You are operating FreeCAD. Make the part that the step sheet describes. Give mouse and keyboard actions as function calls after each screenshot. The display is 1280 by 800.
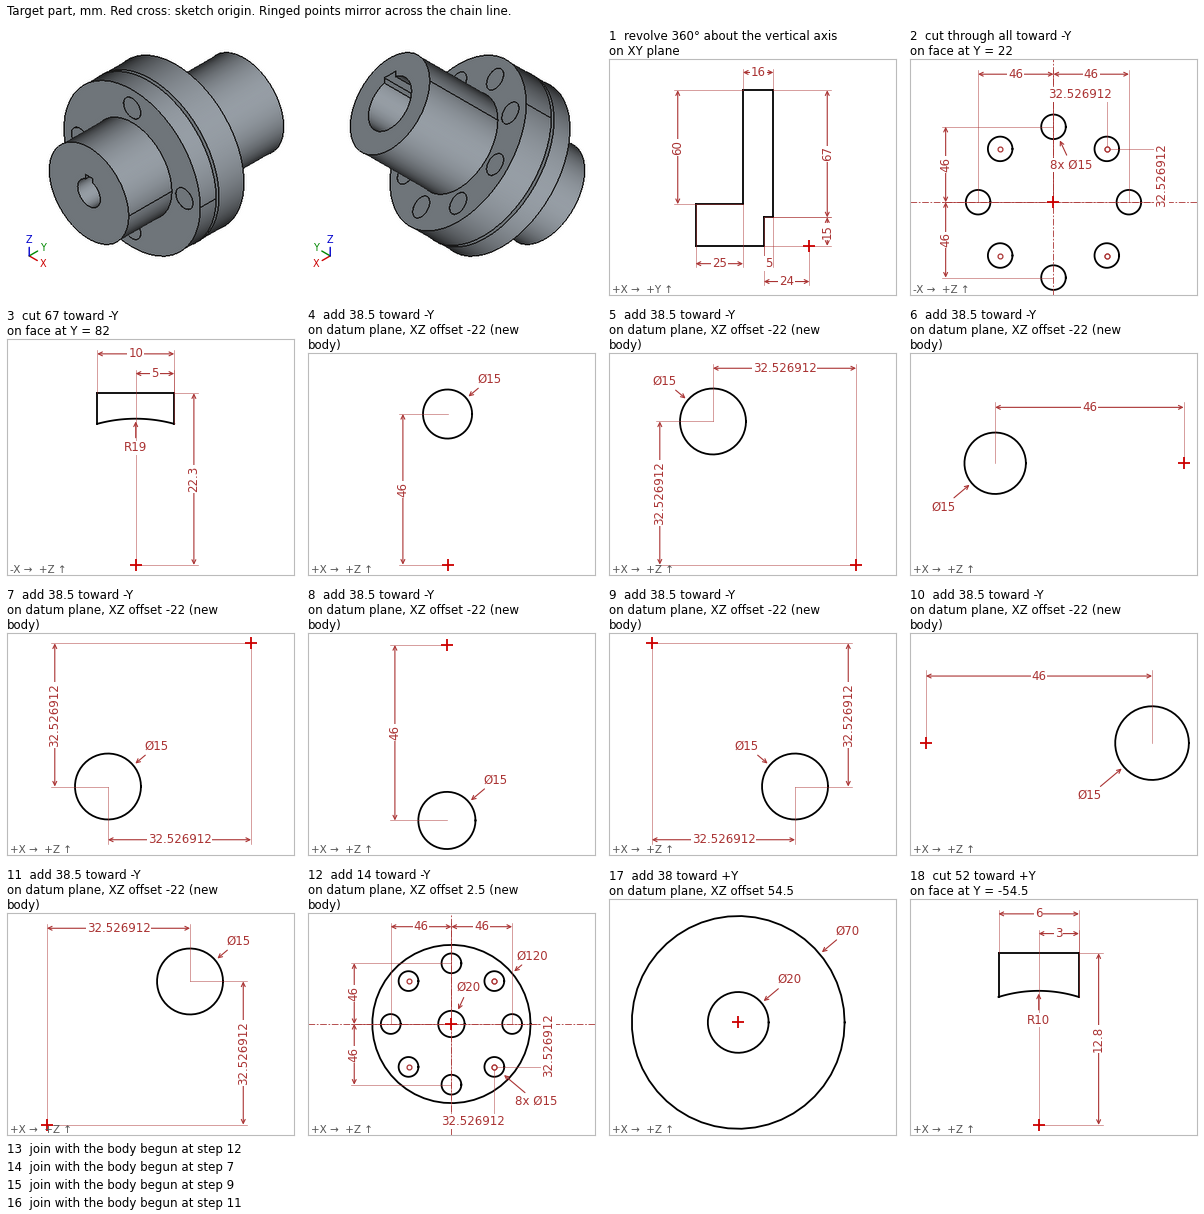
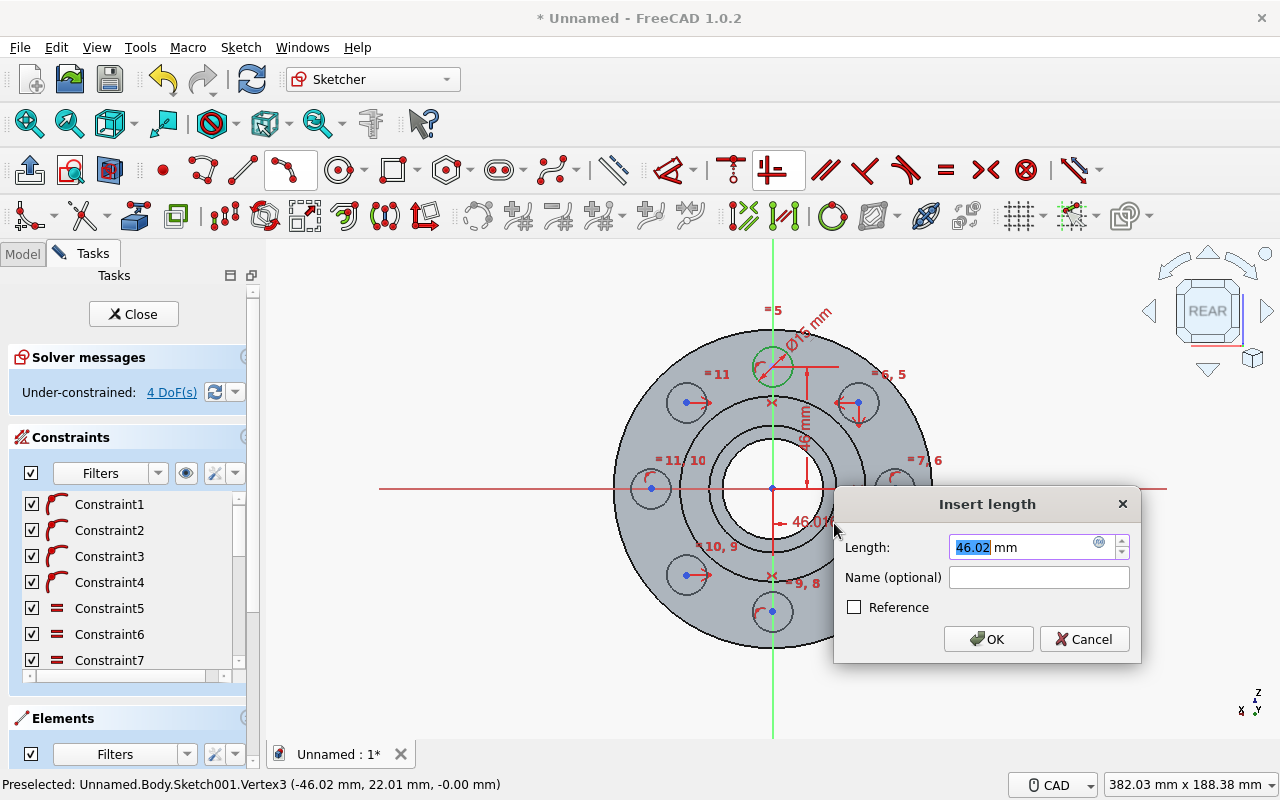
text(46)
key(Return)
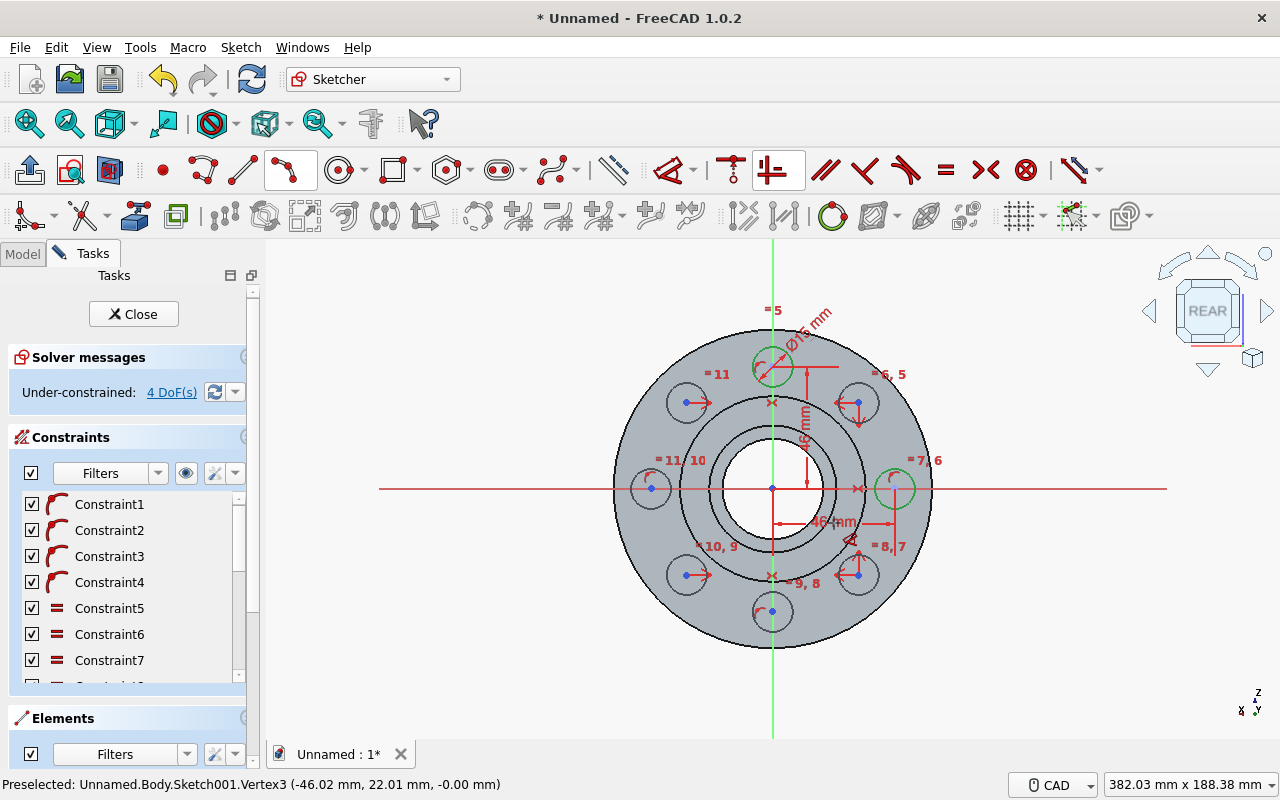
click(773, 612)
click(807, 550)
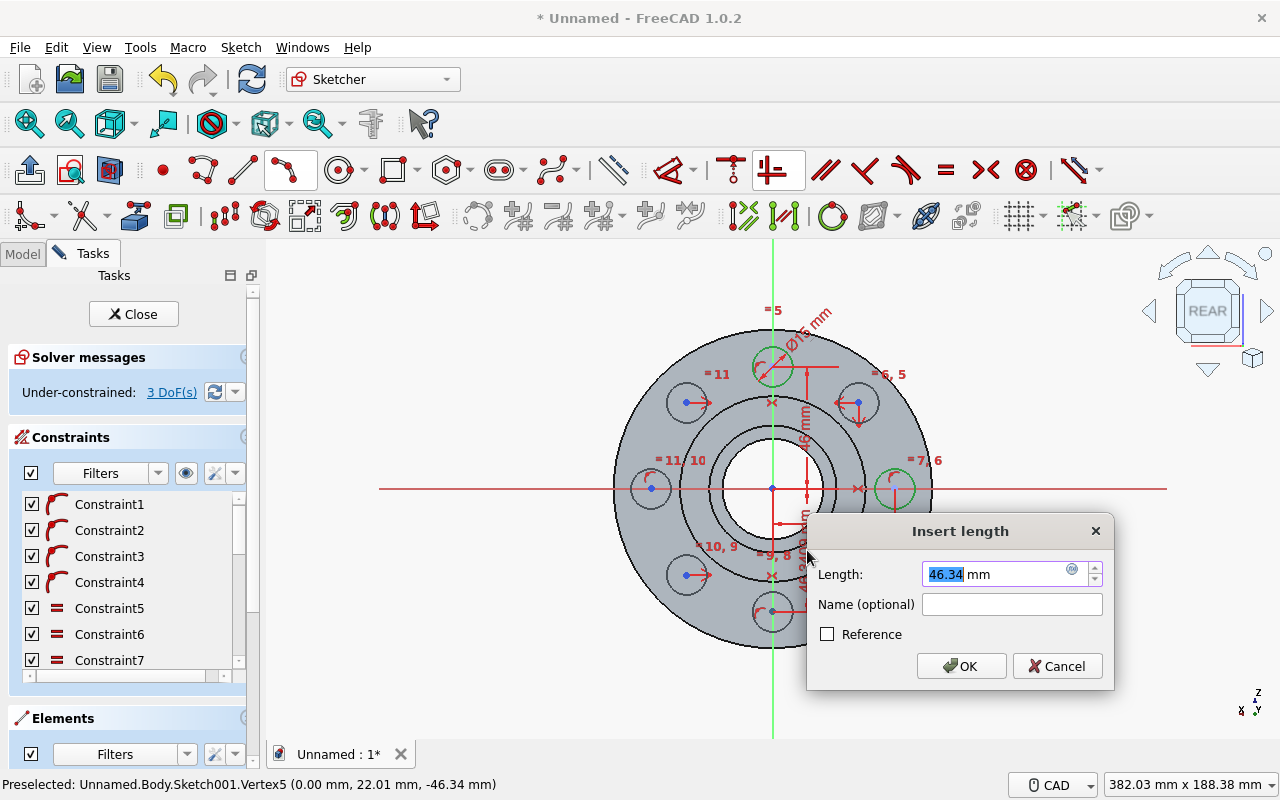
text(46)
key(Return)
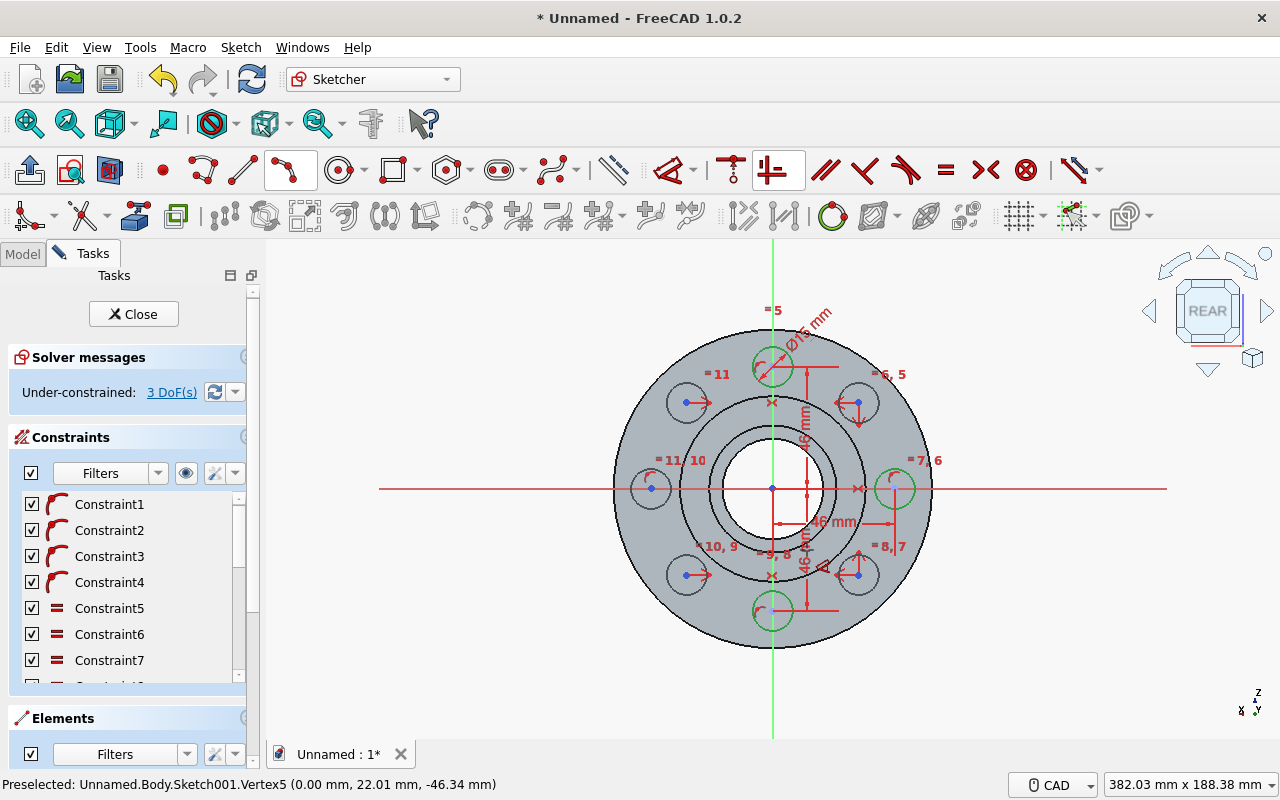
click(651, 489)
click(712, 523)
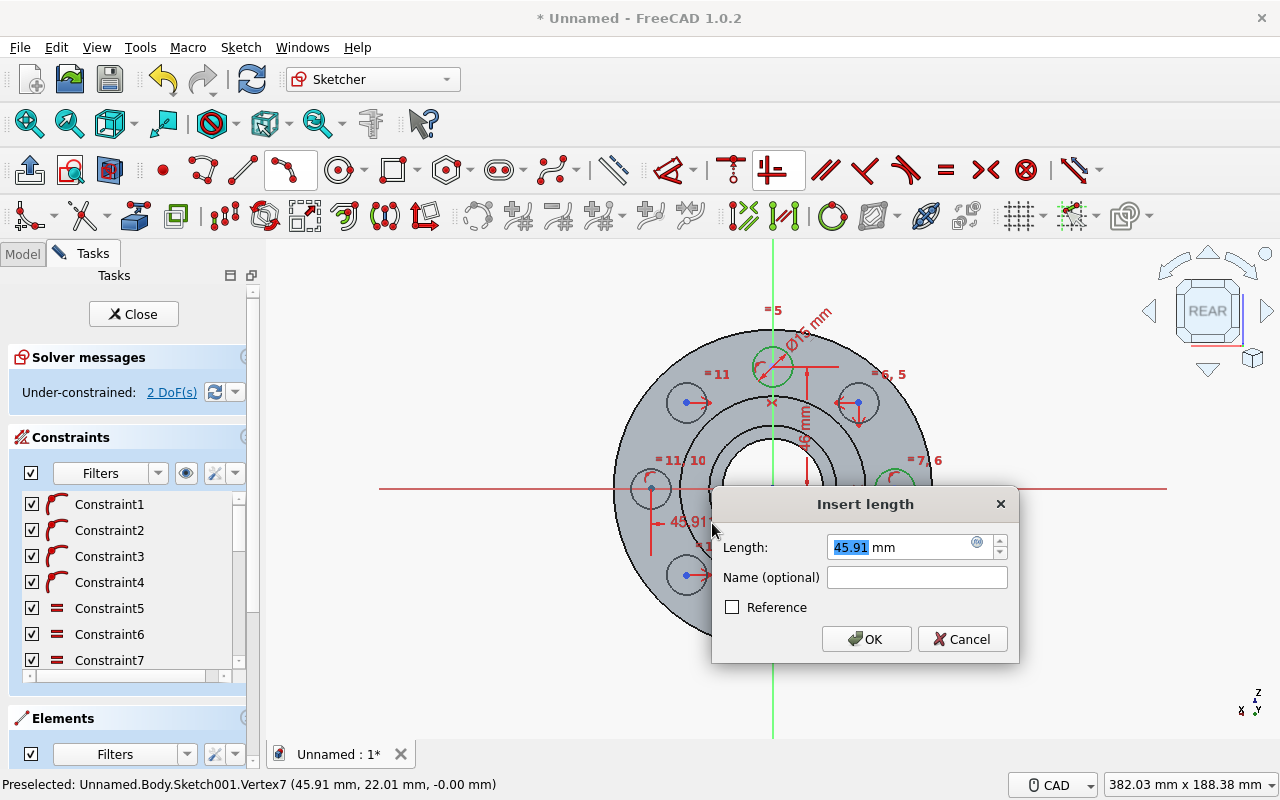
text(46)
key(Return)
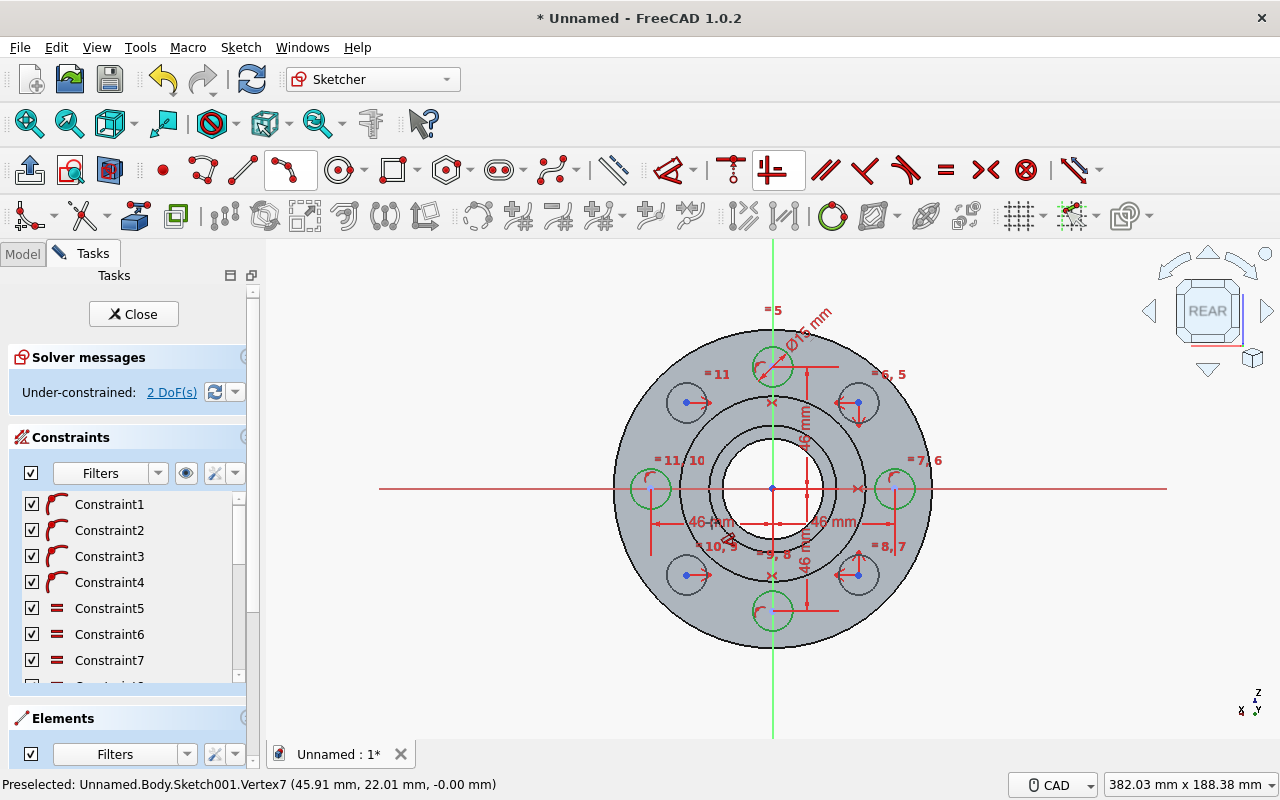
click(859, 403)
click(816, 369)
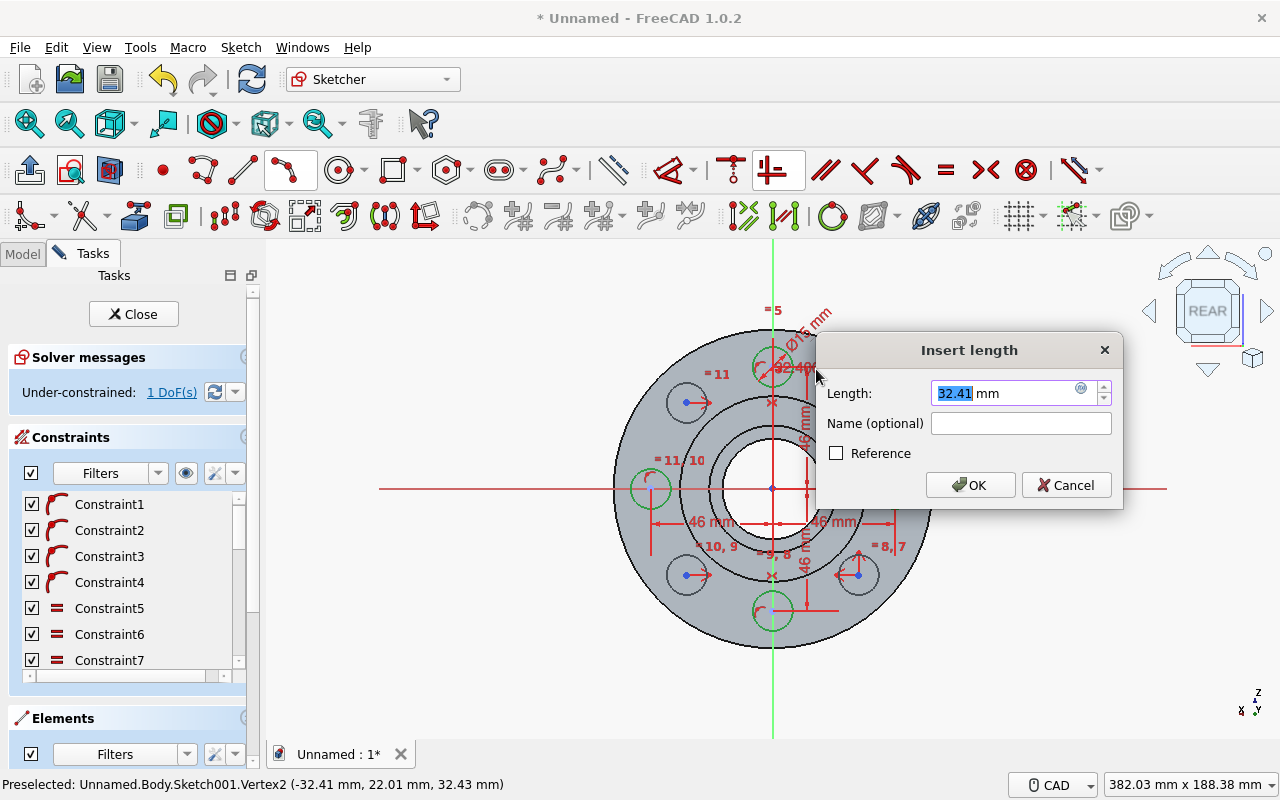
text(32.526912)
key(Return)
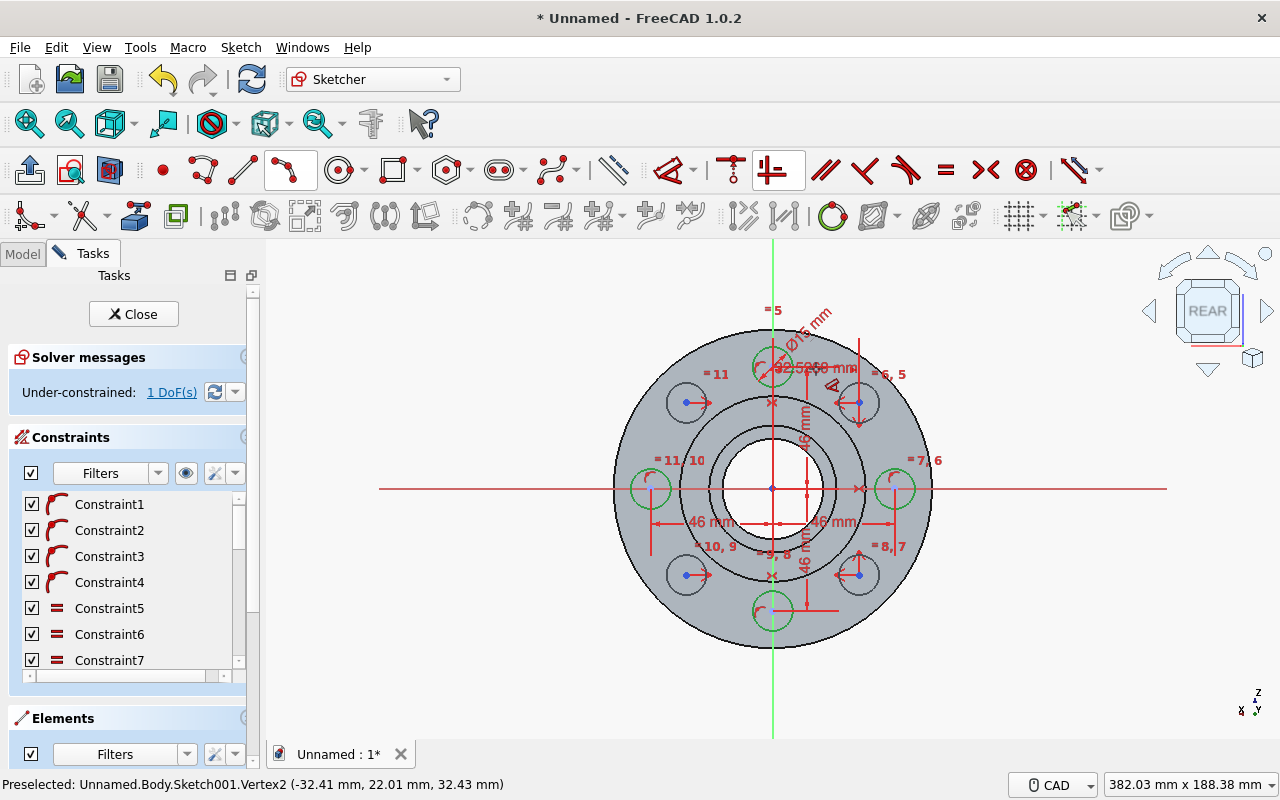
click(859, 403)
click(893, 446)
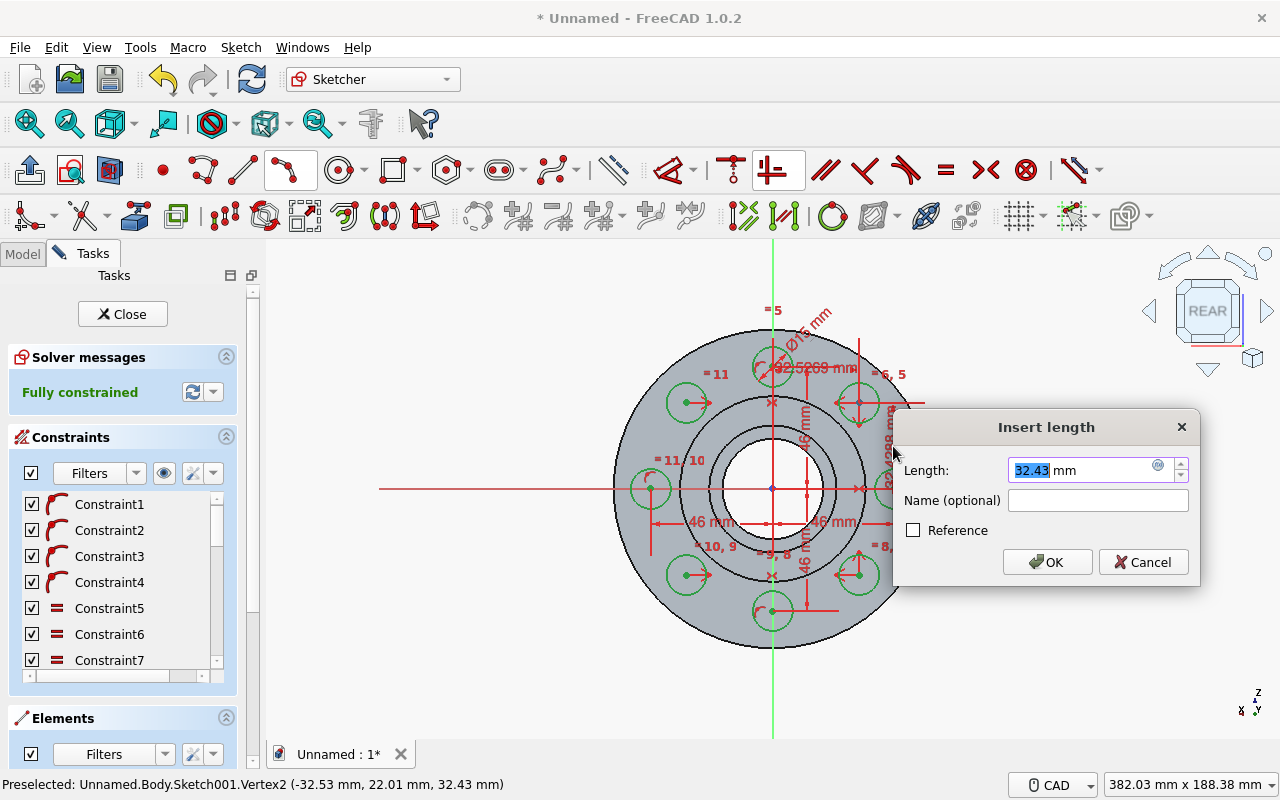
text(32.526912)
key(Return)
key(Escape)